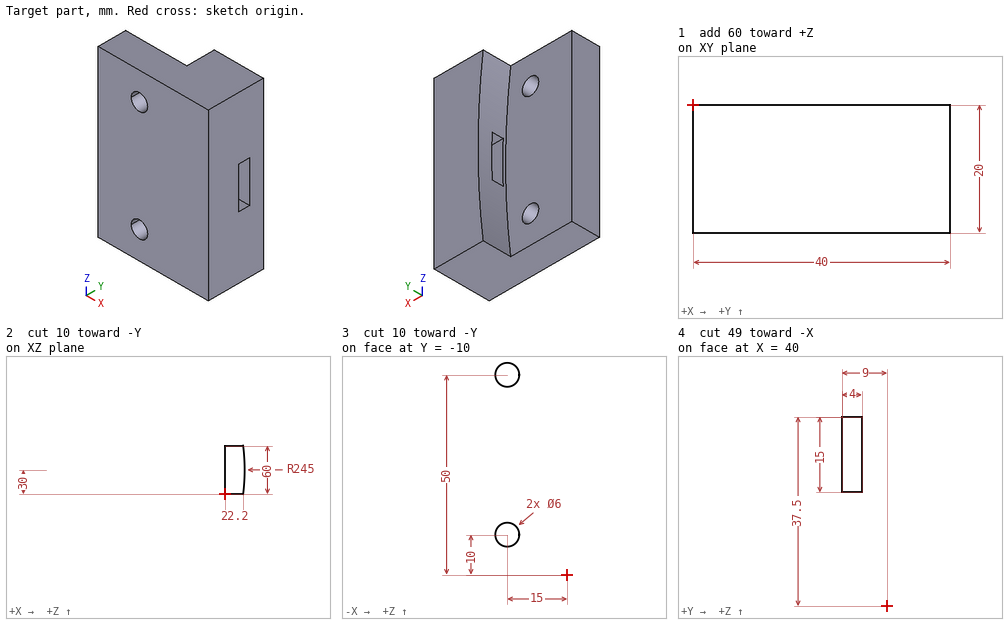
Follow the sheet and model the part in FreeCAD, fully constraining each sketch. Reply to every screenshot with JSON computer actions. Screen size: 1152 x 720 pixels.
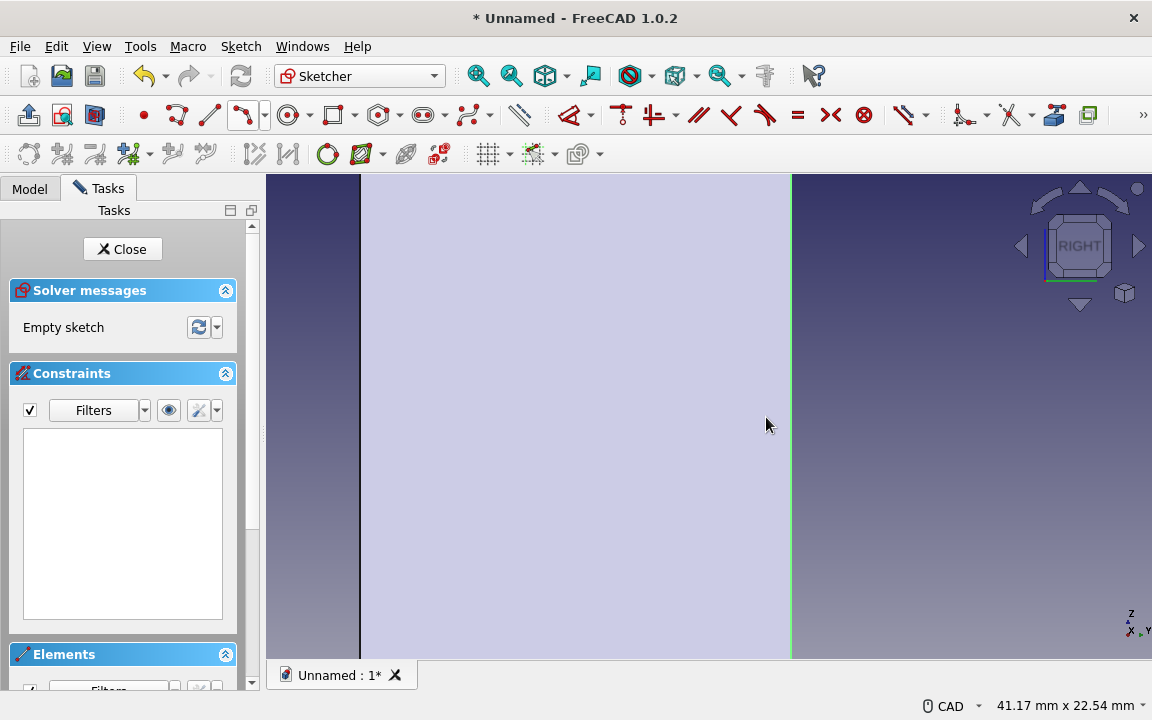
{"action": "left_click", "coordinate": [332, 116]}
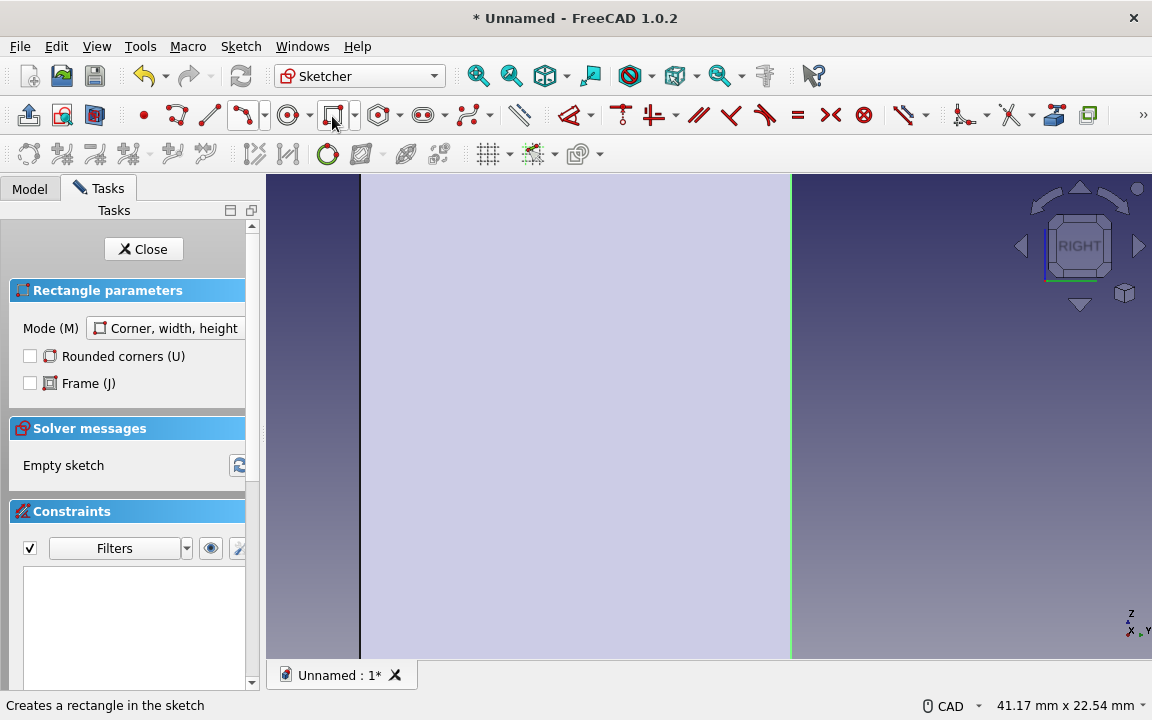
{"action": "left_click", "coordinate": [597, 253]}
{"action": "mouse_move", "coordinate": [683, 576]}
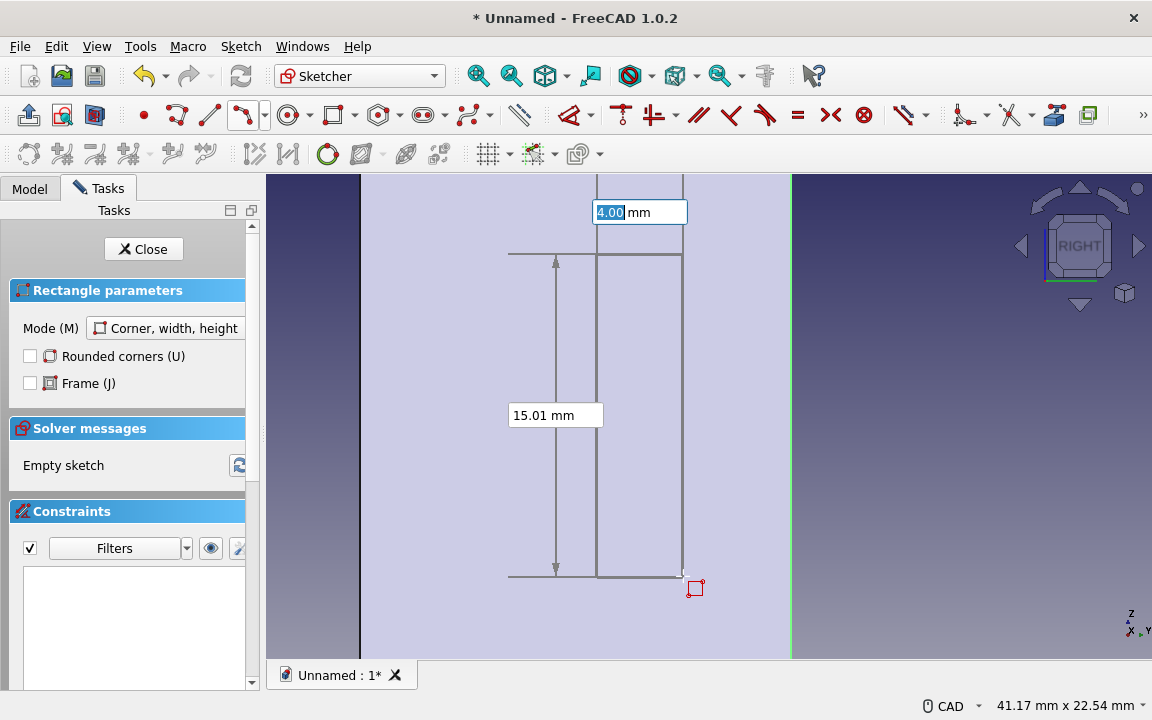
{"action": "type", "text": "4"}
{"action": "key", "text": "Tab"}
{"action": "type", "text": "15"}
{"action": "key", "text": "Return"}
{"action": "key", "text": "Escape"}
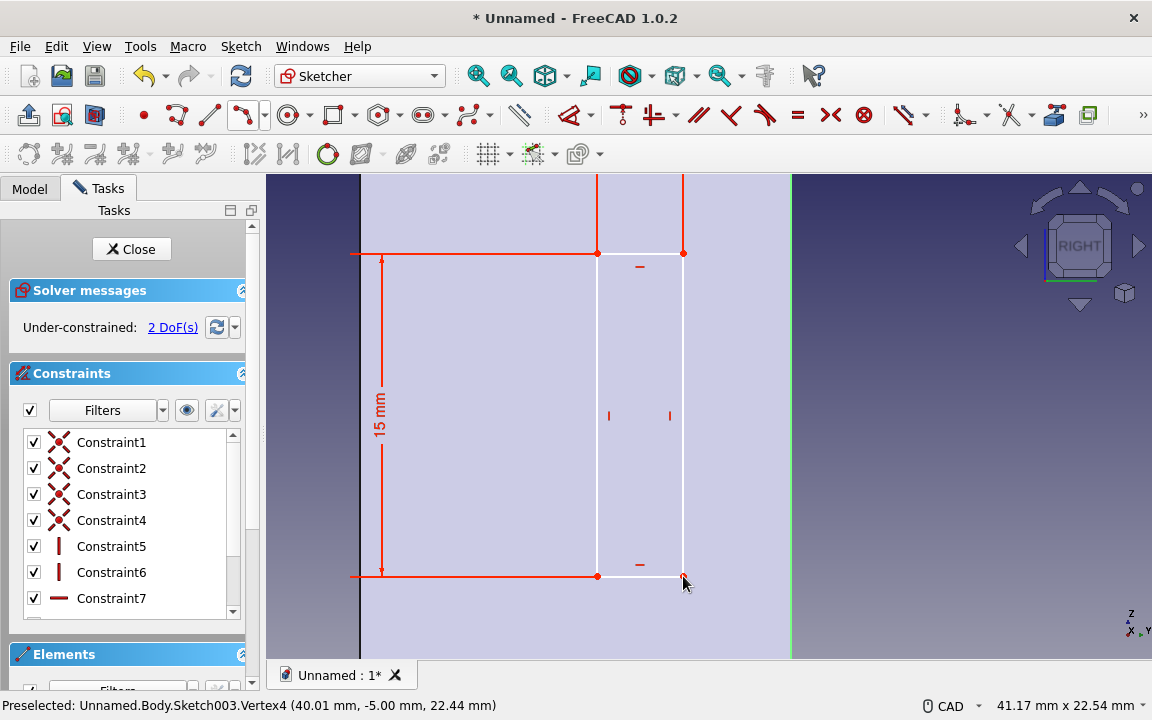
{"action": "left_click", "coordinate": [568, 116]}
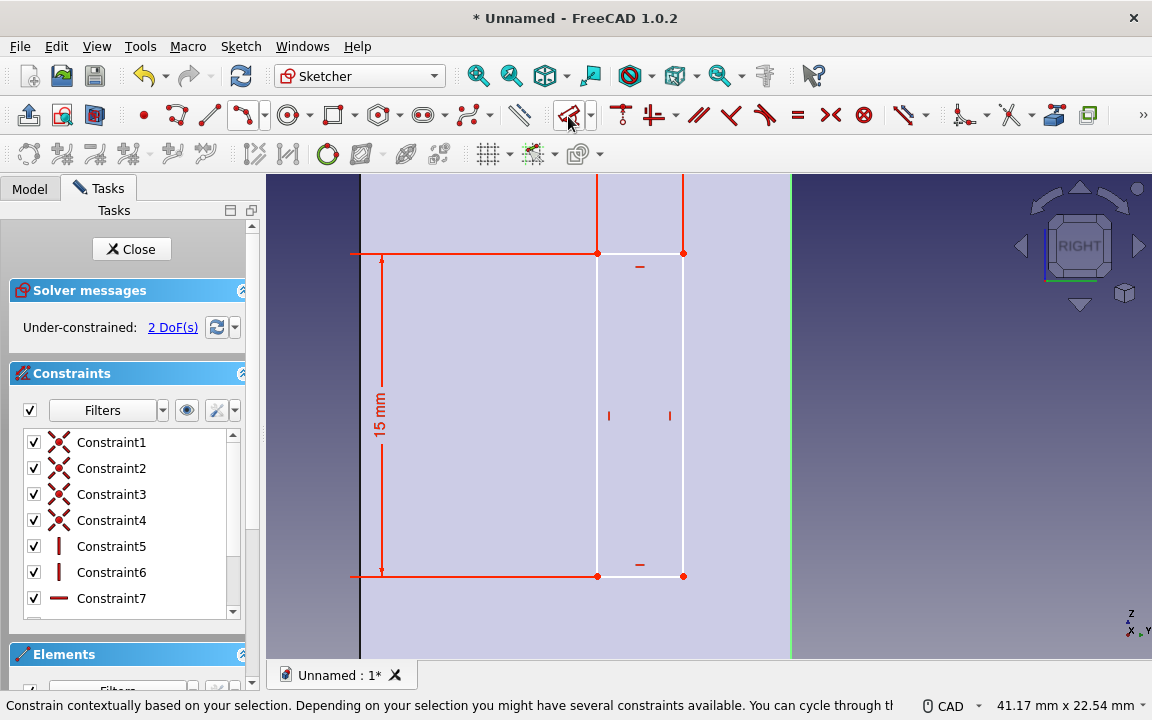
{"action": "left_click", "coordinate": [597, 254]}
{"action": "left_click", "coordinate": [694, 220]}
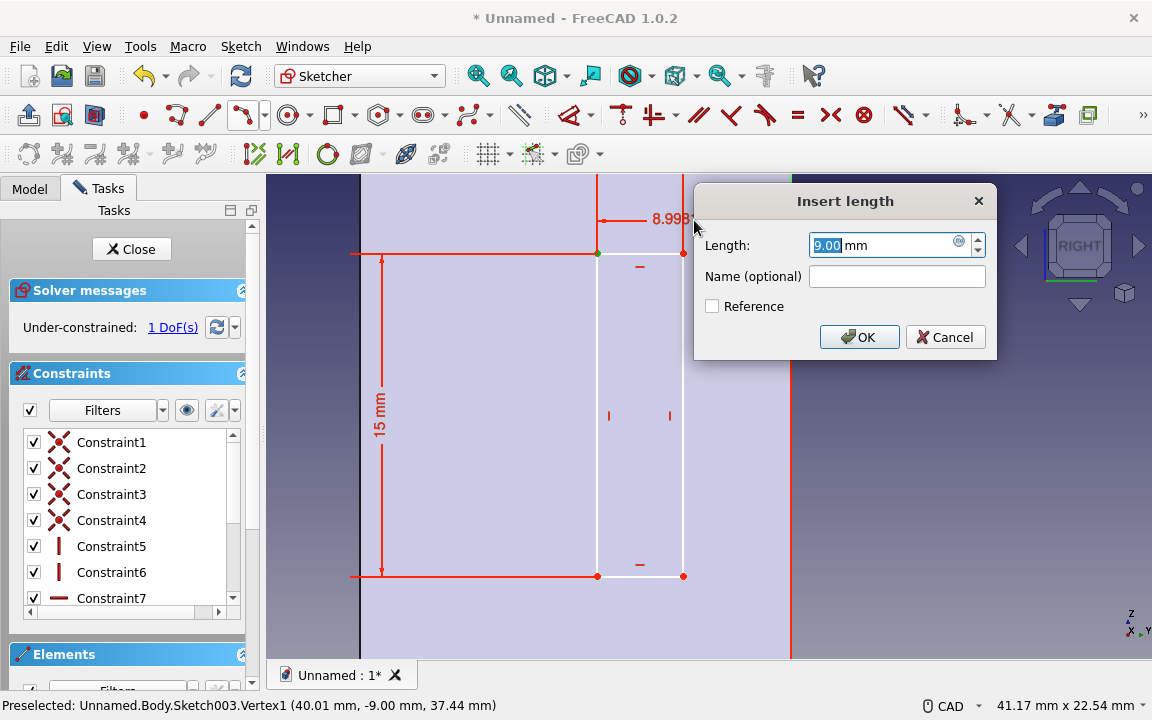
{"action": "type", "text": "9"}
{"action": "key", "text": "Return"}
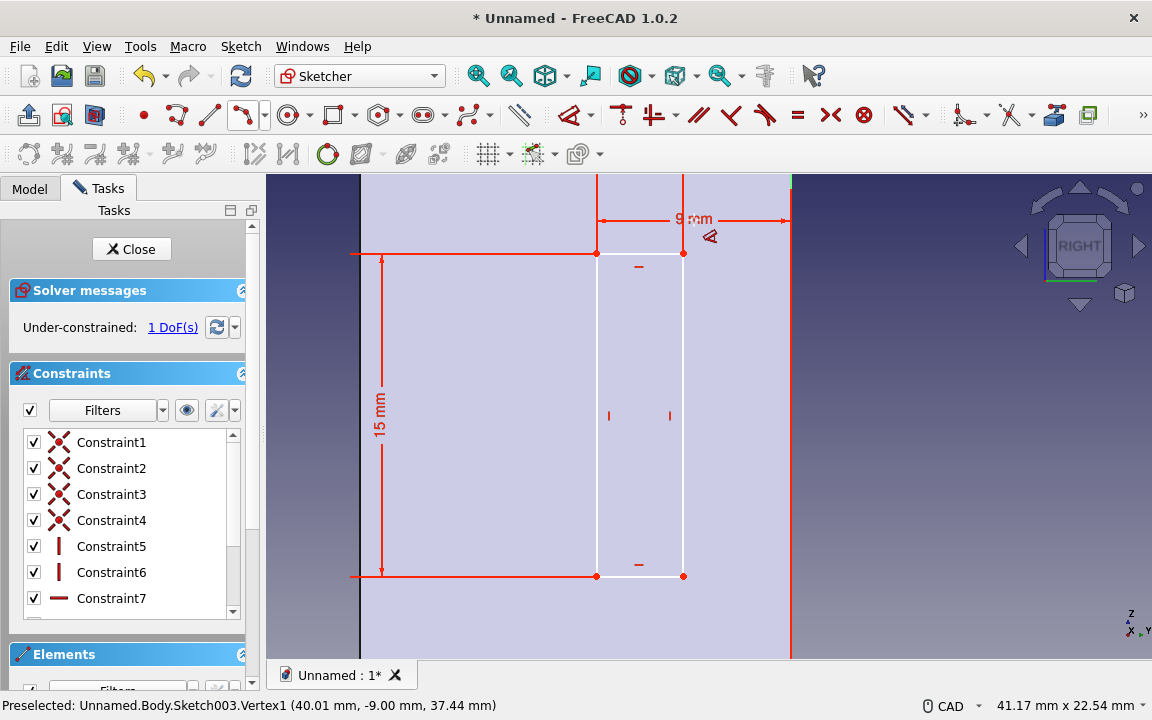
{"action": "left_click", "coordinate": [597, 254]}
{"action": "left_click", "coordinate": [825, 443]}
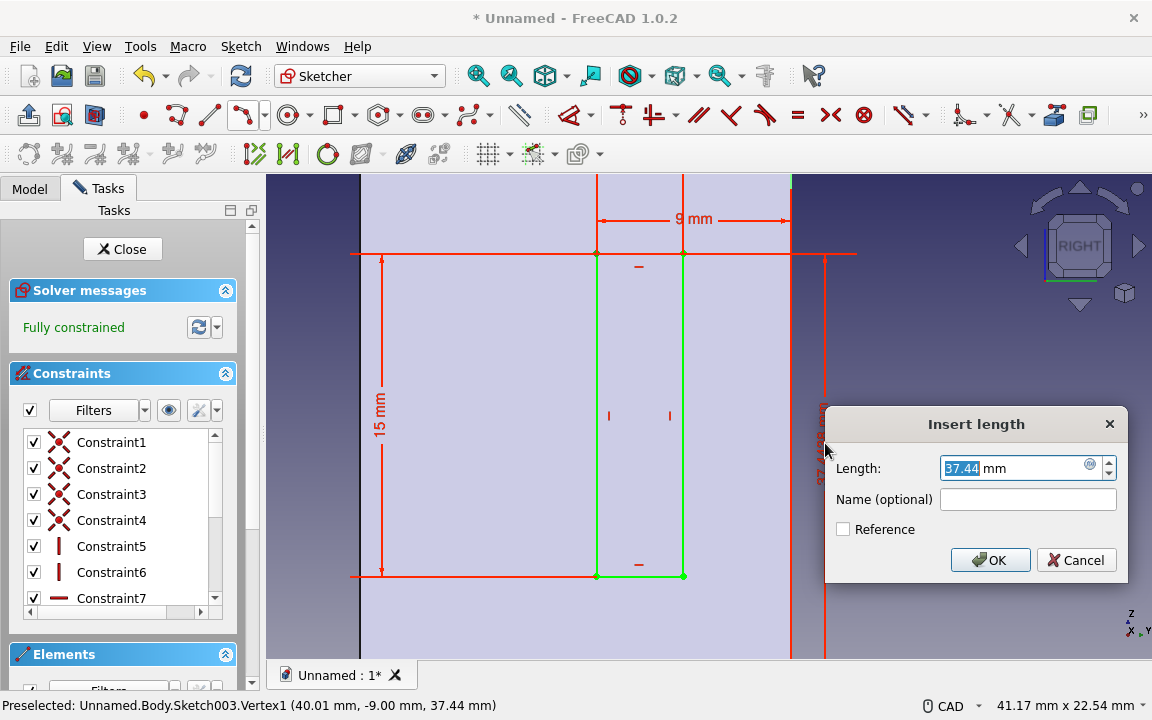
{"action": "type", "text": "37.5"}
{"action": "key", "text": "Return"}
{"action": "key", "text": "Escape"}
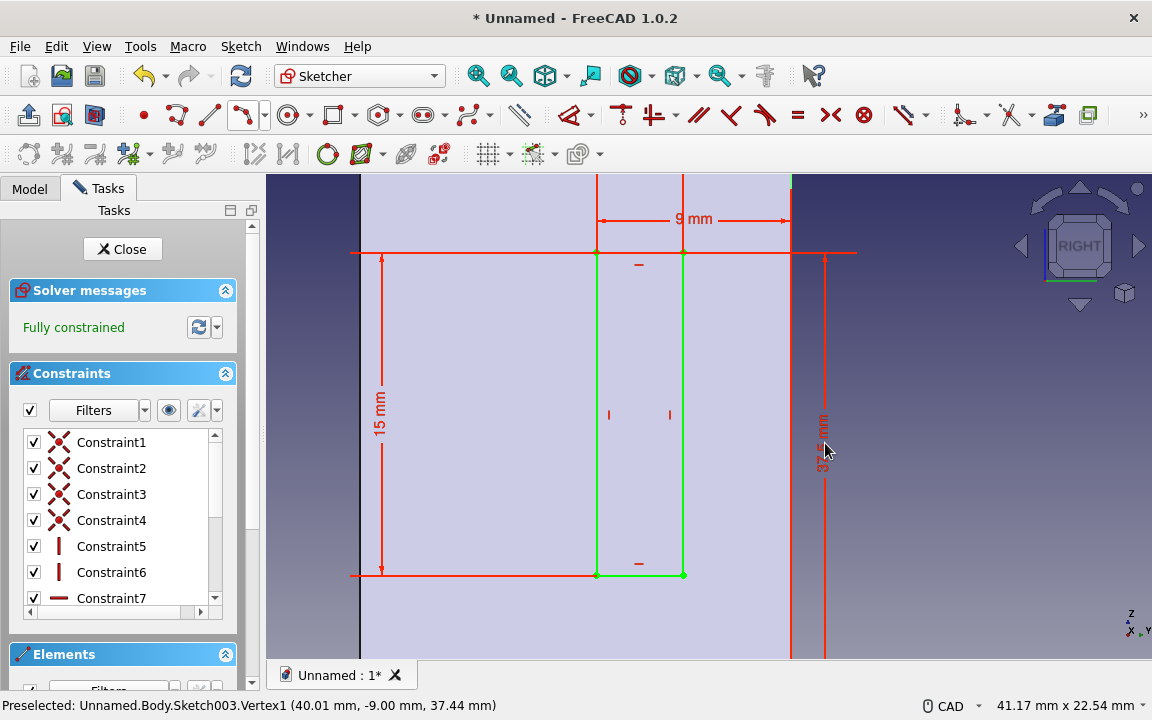
{"action": "left_click", "coordinate": [123, 249]}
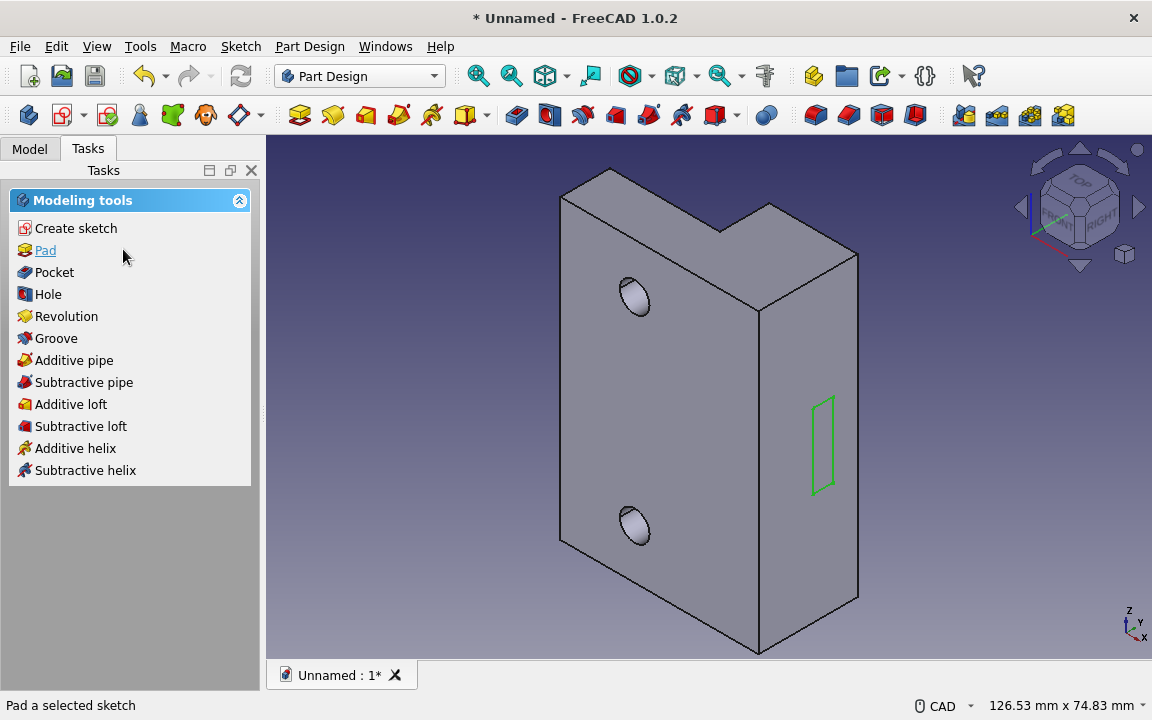
{"action": "left_click", "coordinate": [517, 116]}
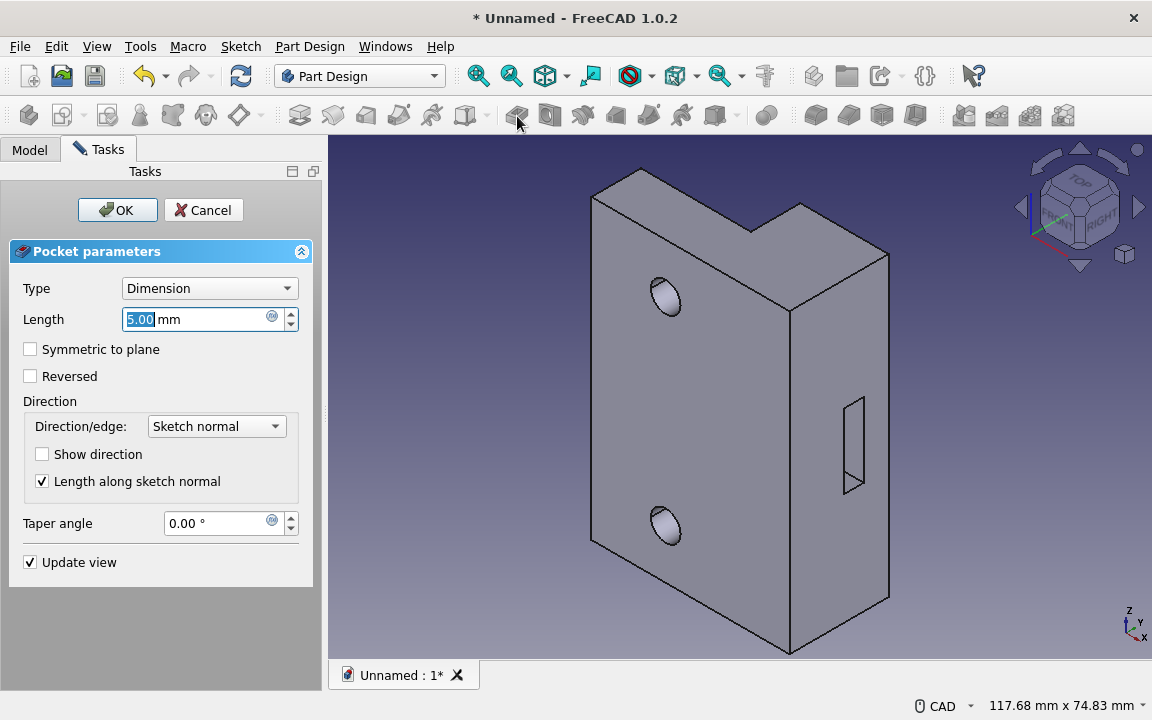
{"action": "type", "text": "49"}
{"action": "key", "text": "Tab"}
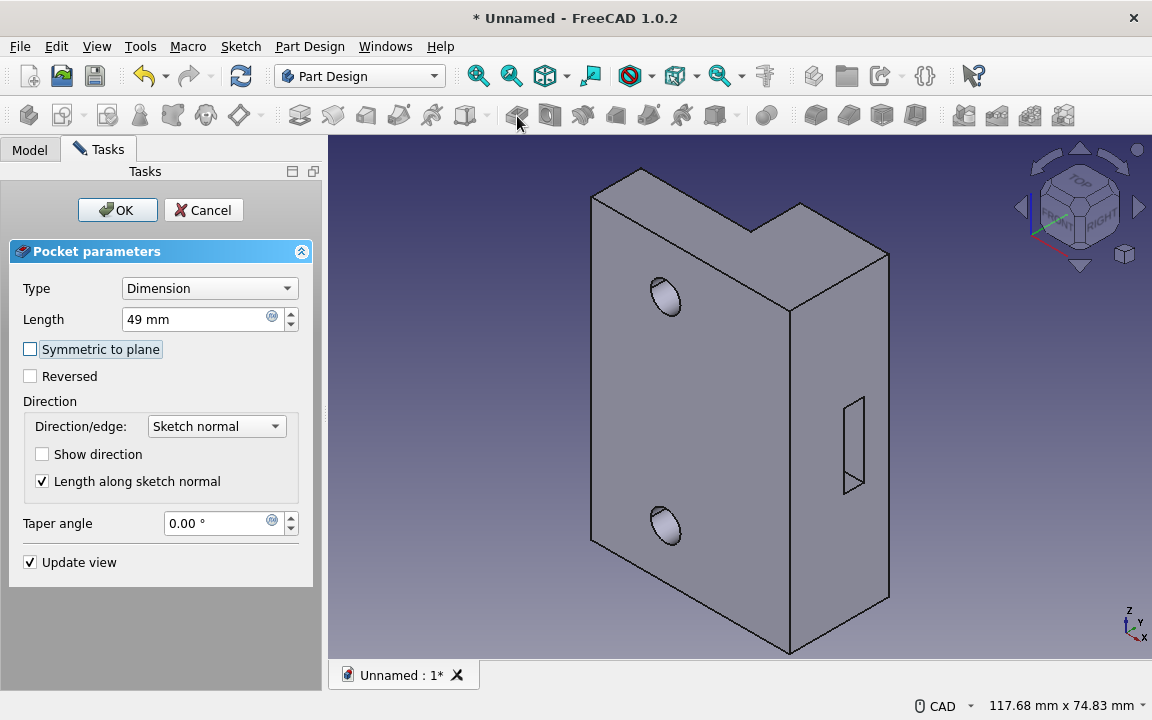
{"action": "left_click", "coordinate": [118, 210]}